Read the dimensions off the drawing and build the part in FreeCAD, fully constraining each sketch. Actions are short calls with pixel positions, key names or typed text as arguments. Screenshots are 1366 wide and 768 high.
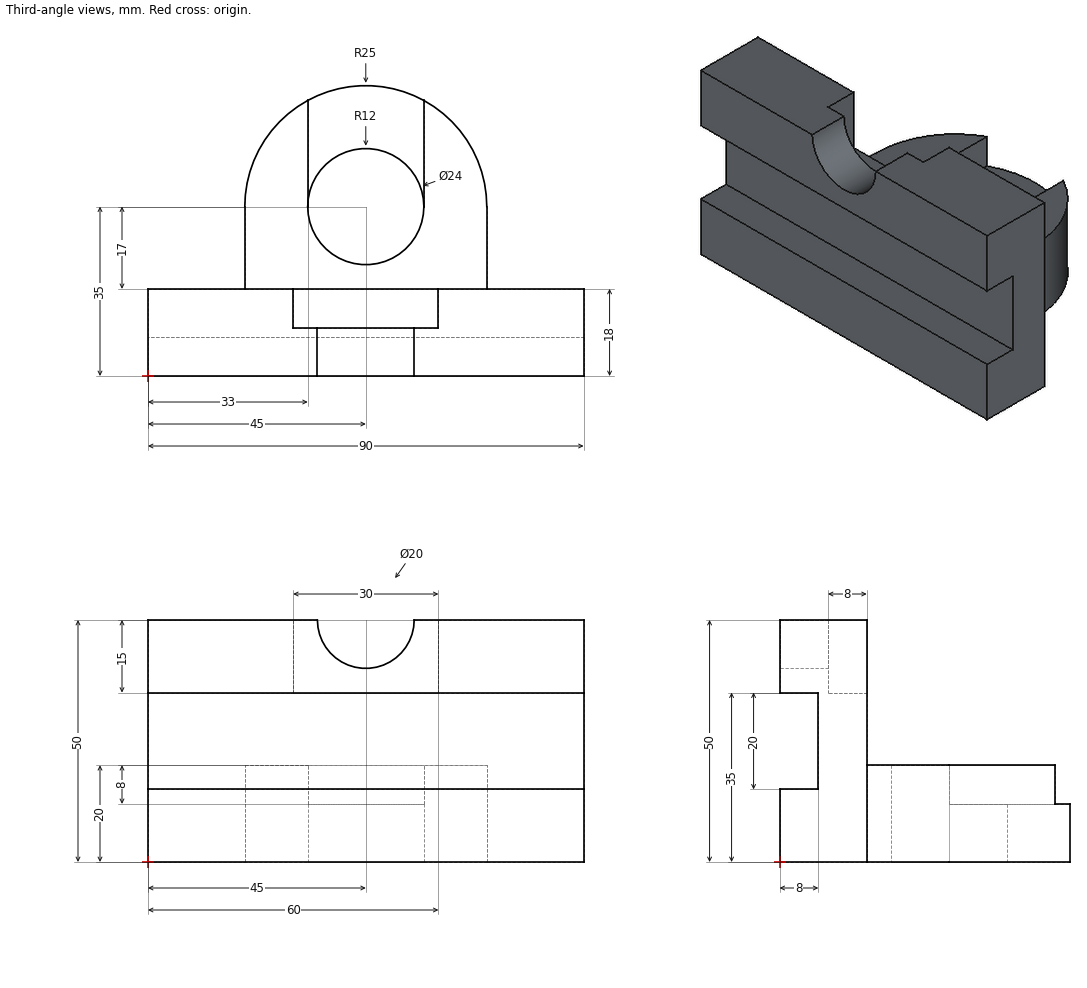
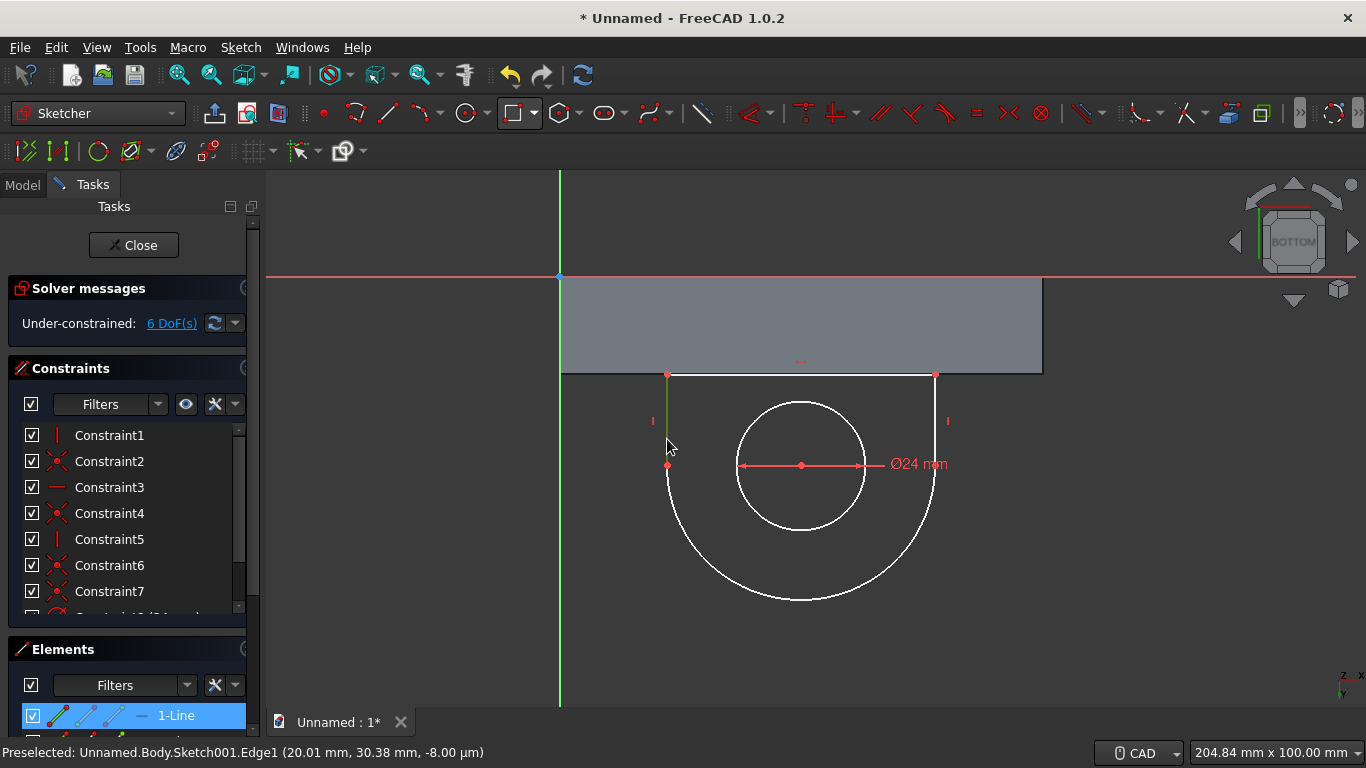
click(722, 574)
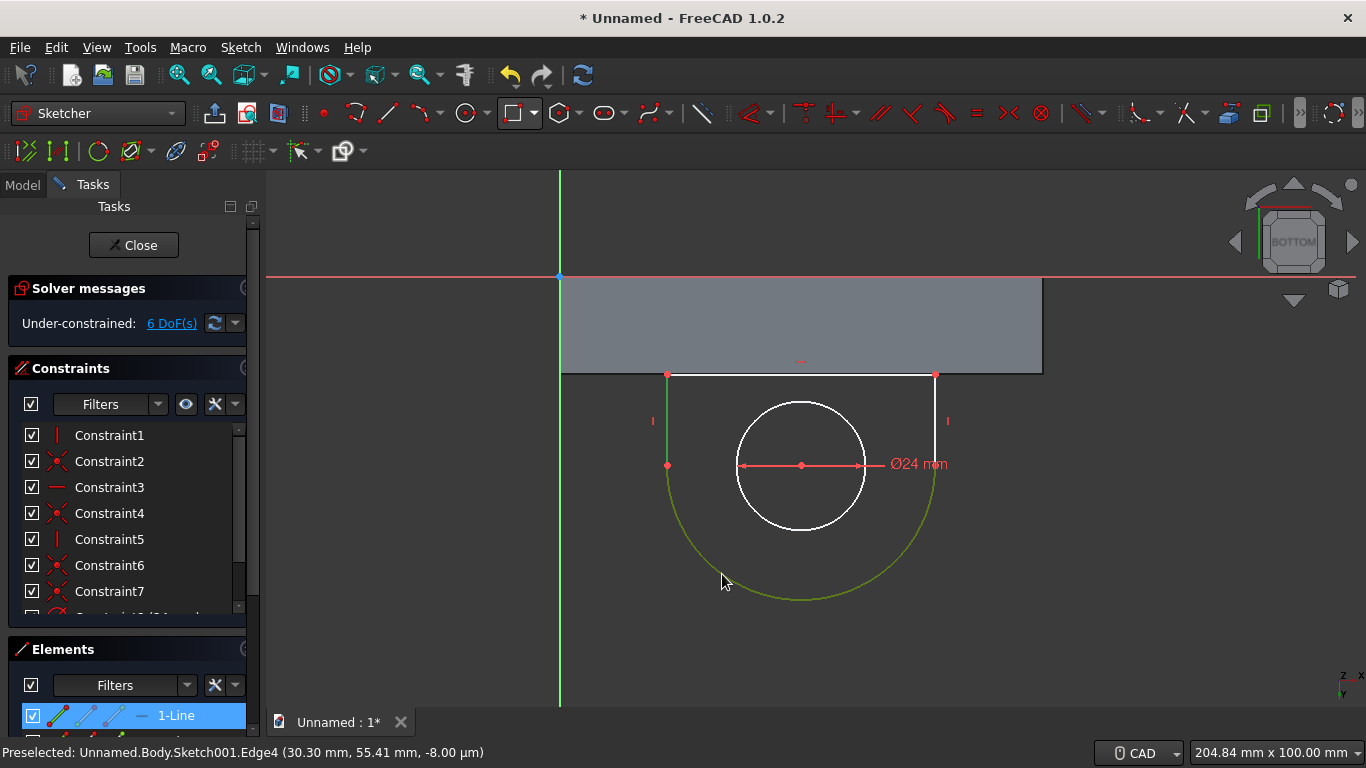
click(946, 114)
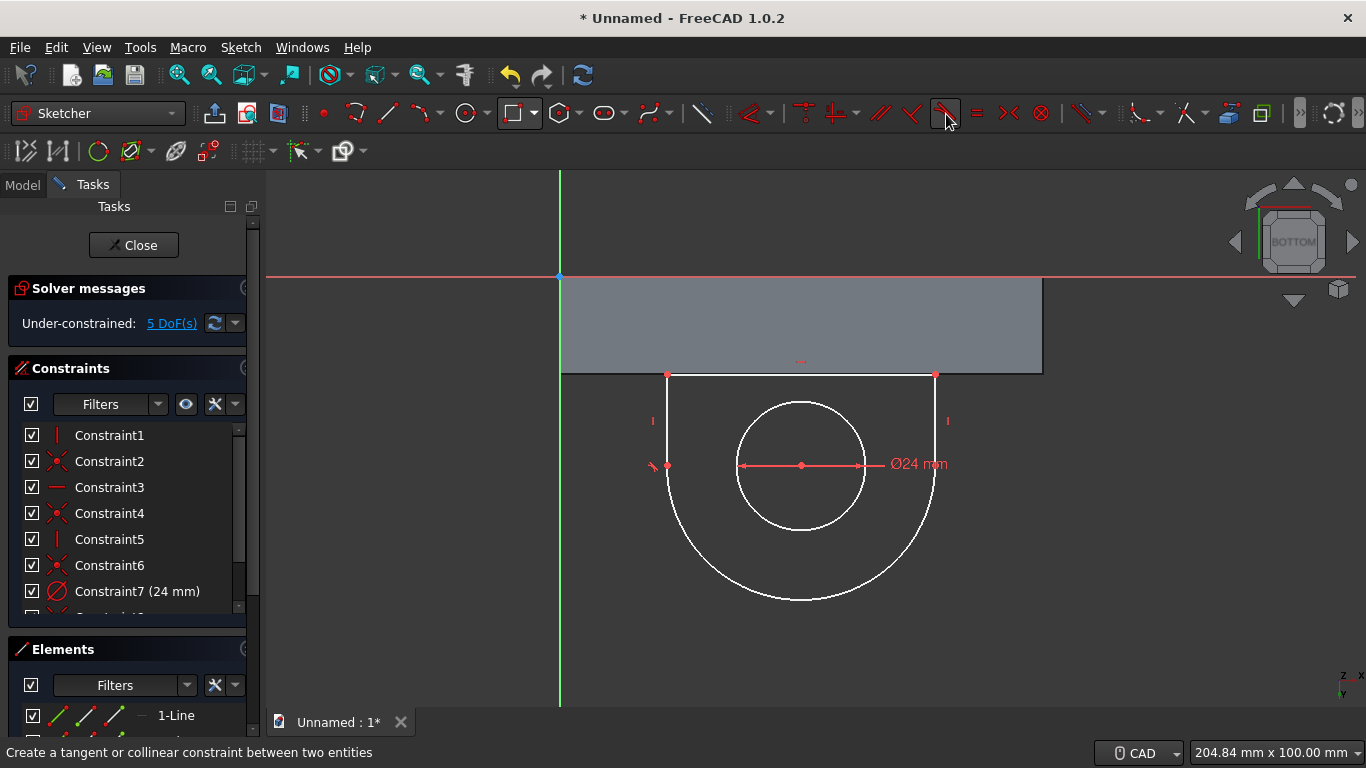
click(935, 402)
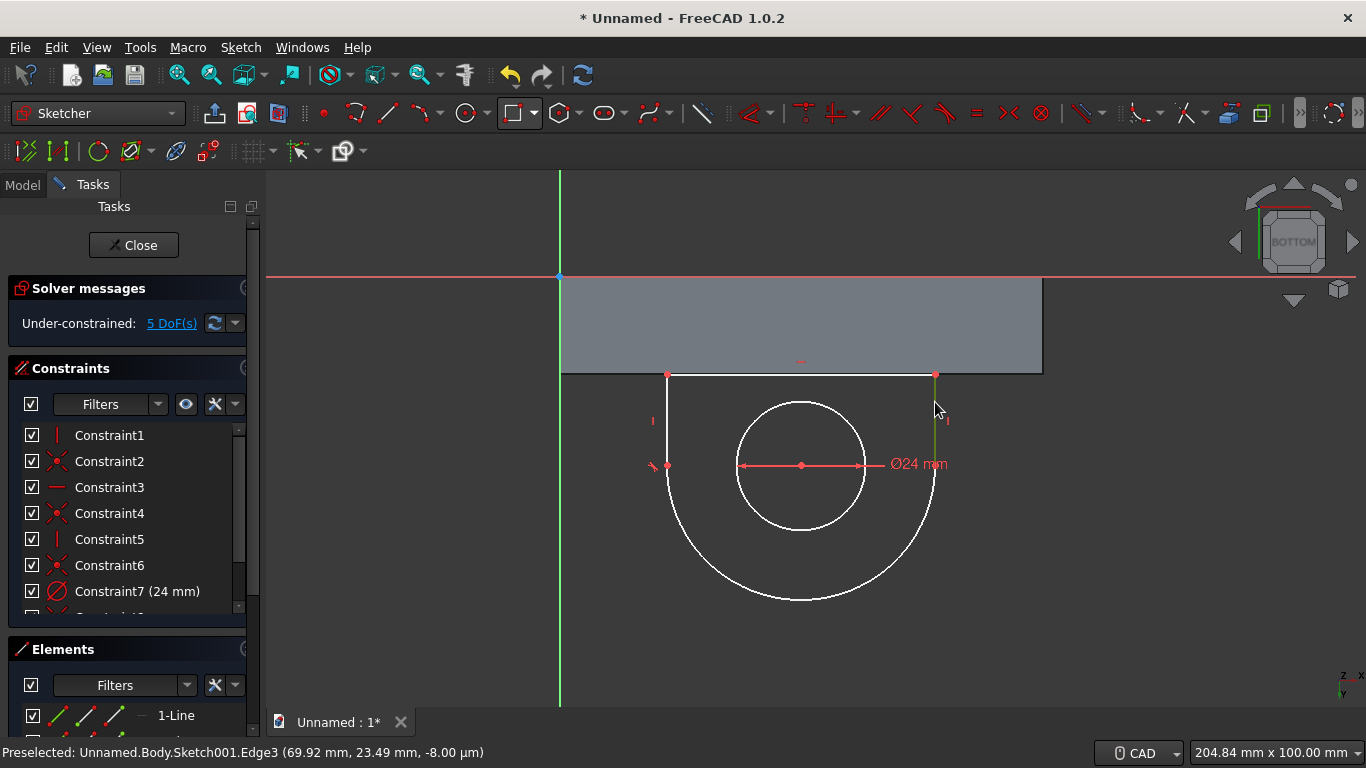
click(722, 574)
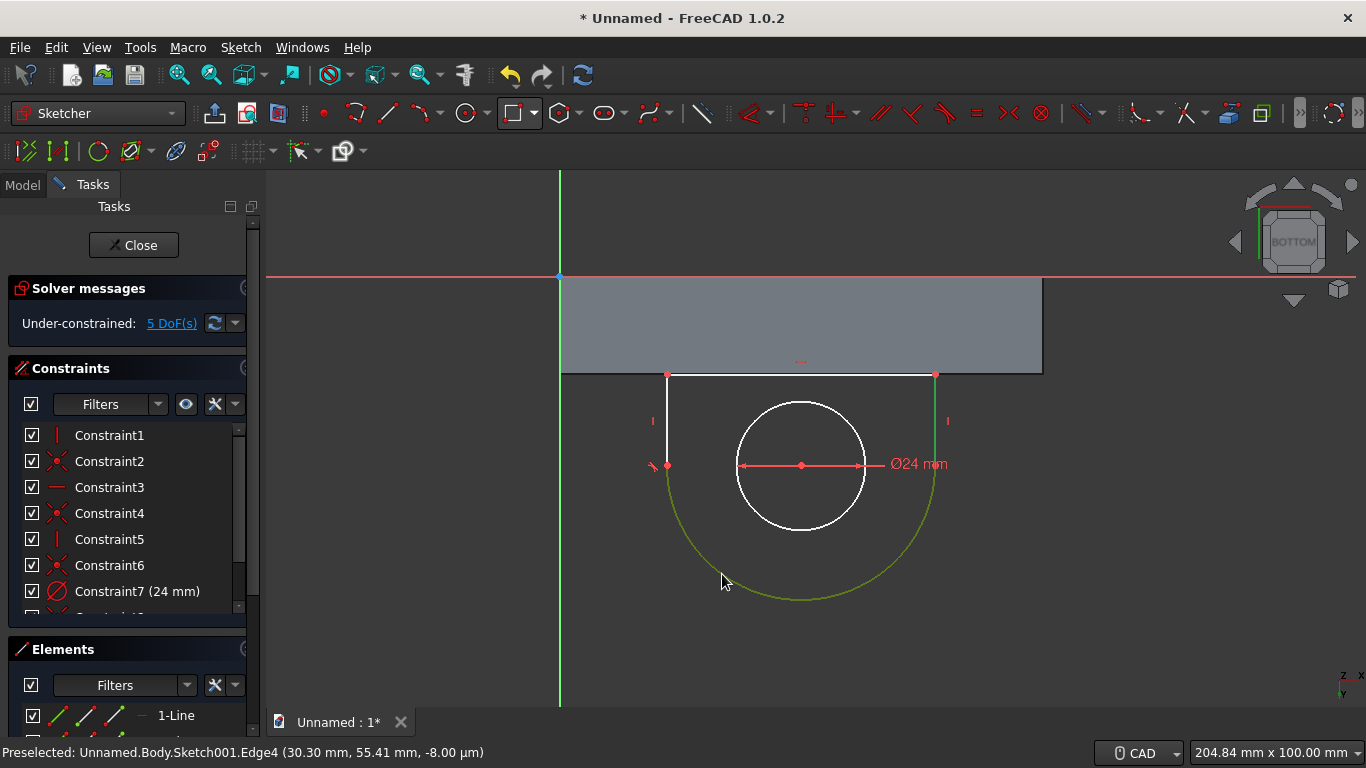
key(t)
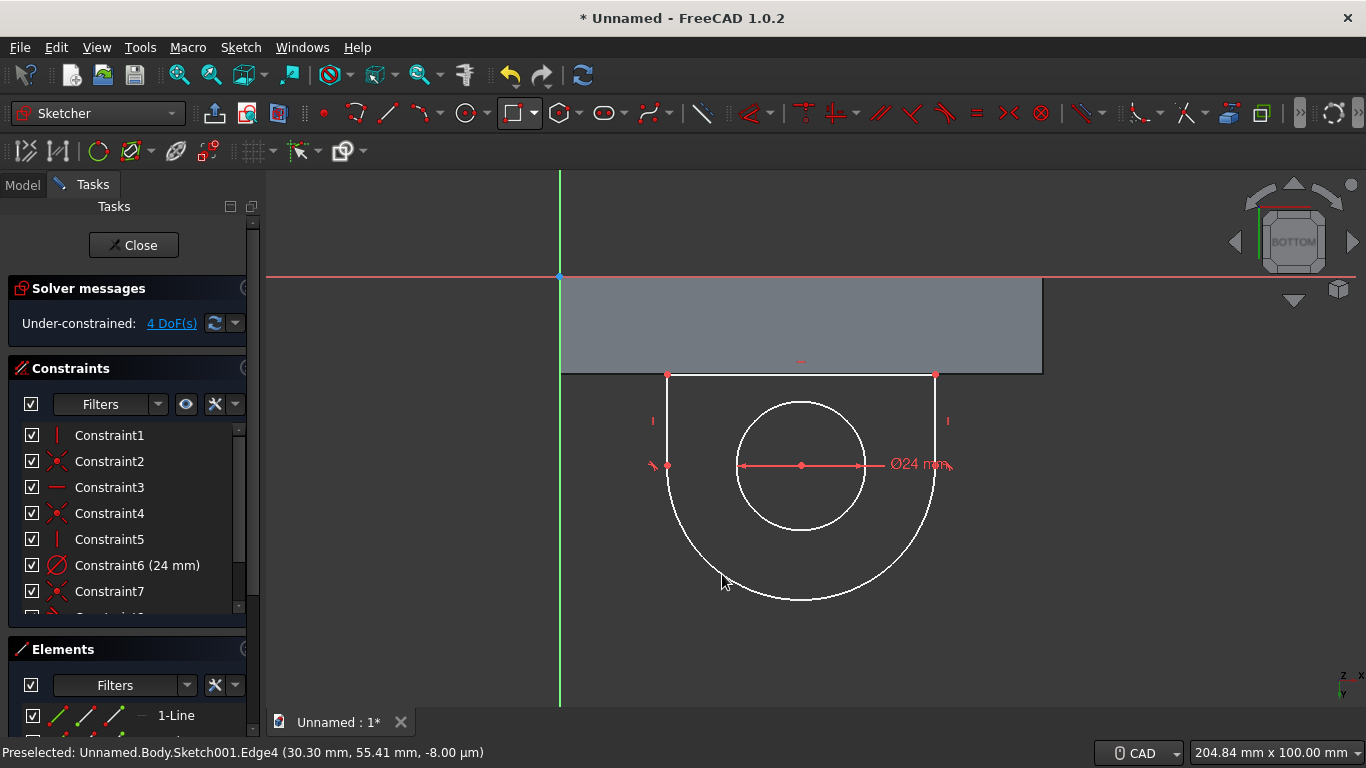
key(d)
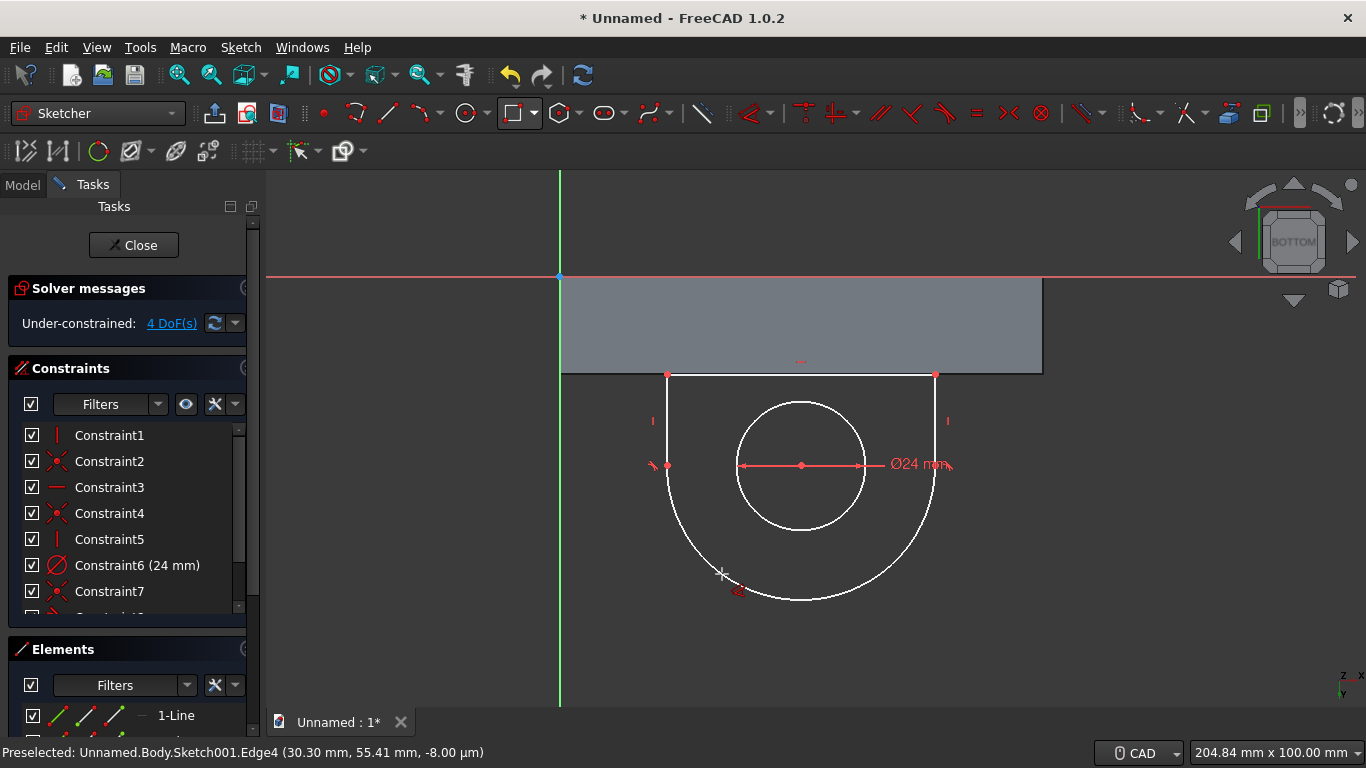
click(722, 574)
click(703, 600)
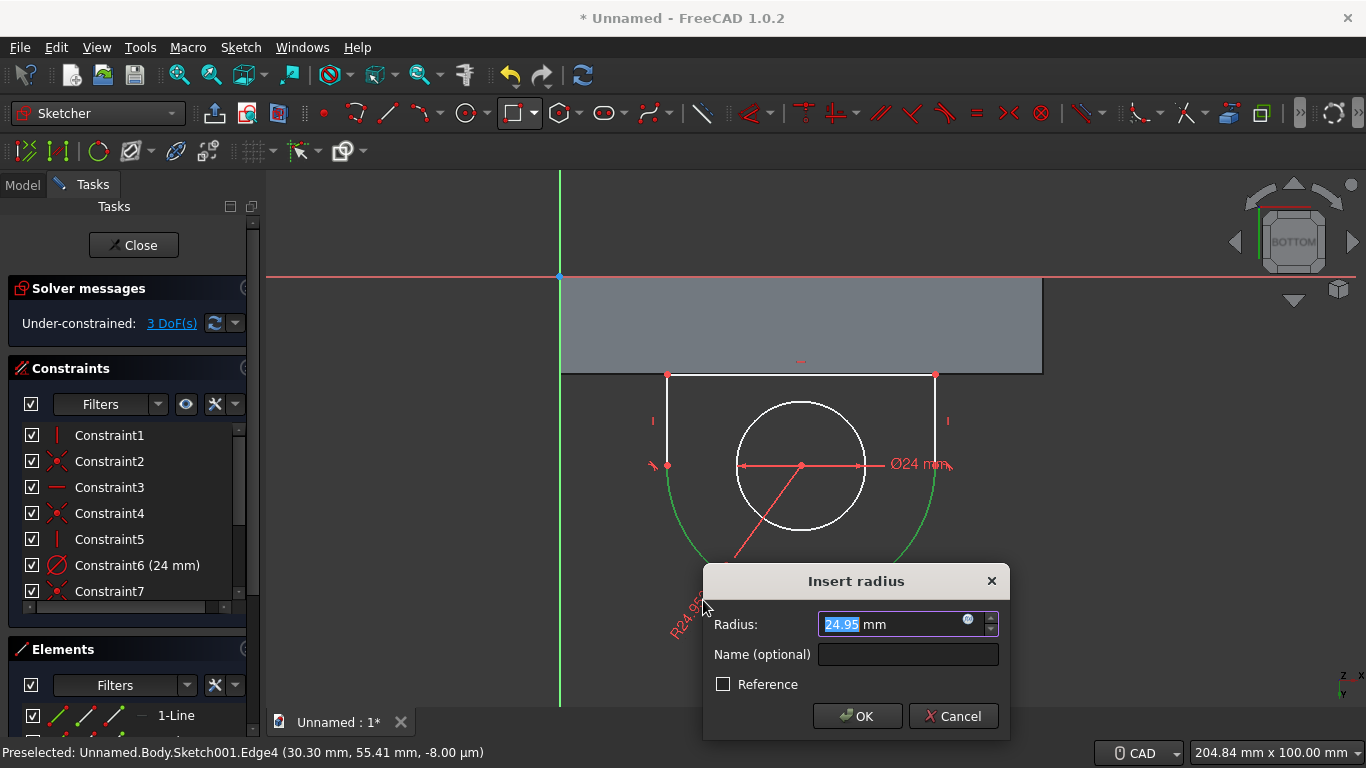
text(25)
key(Return)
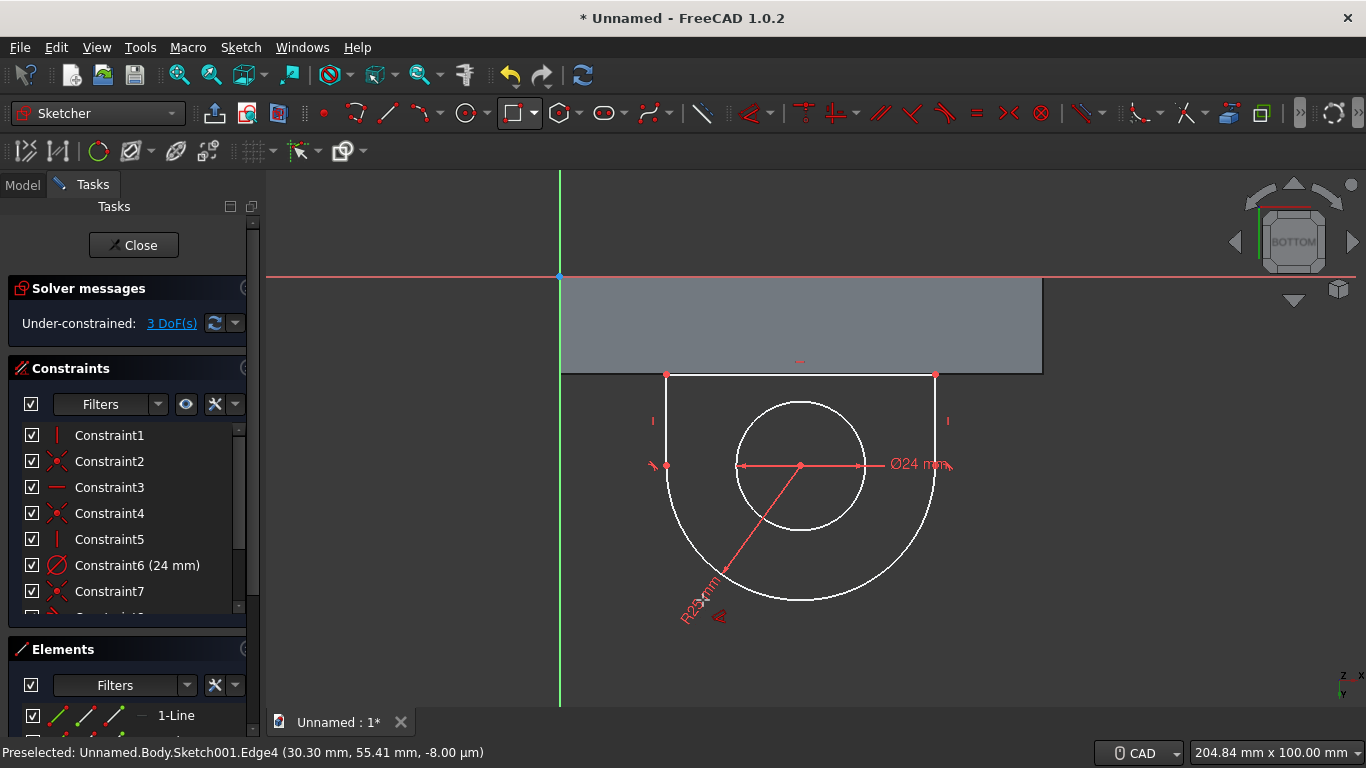
click(666, 439)
click(632, 421)